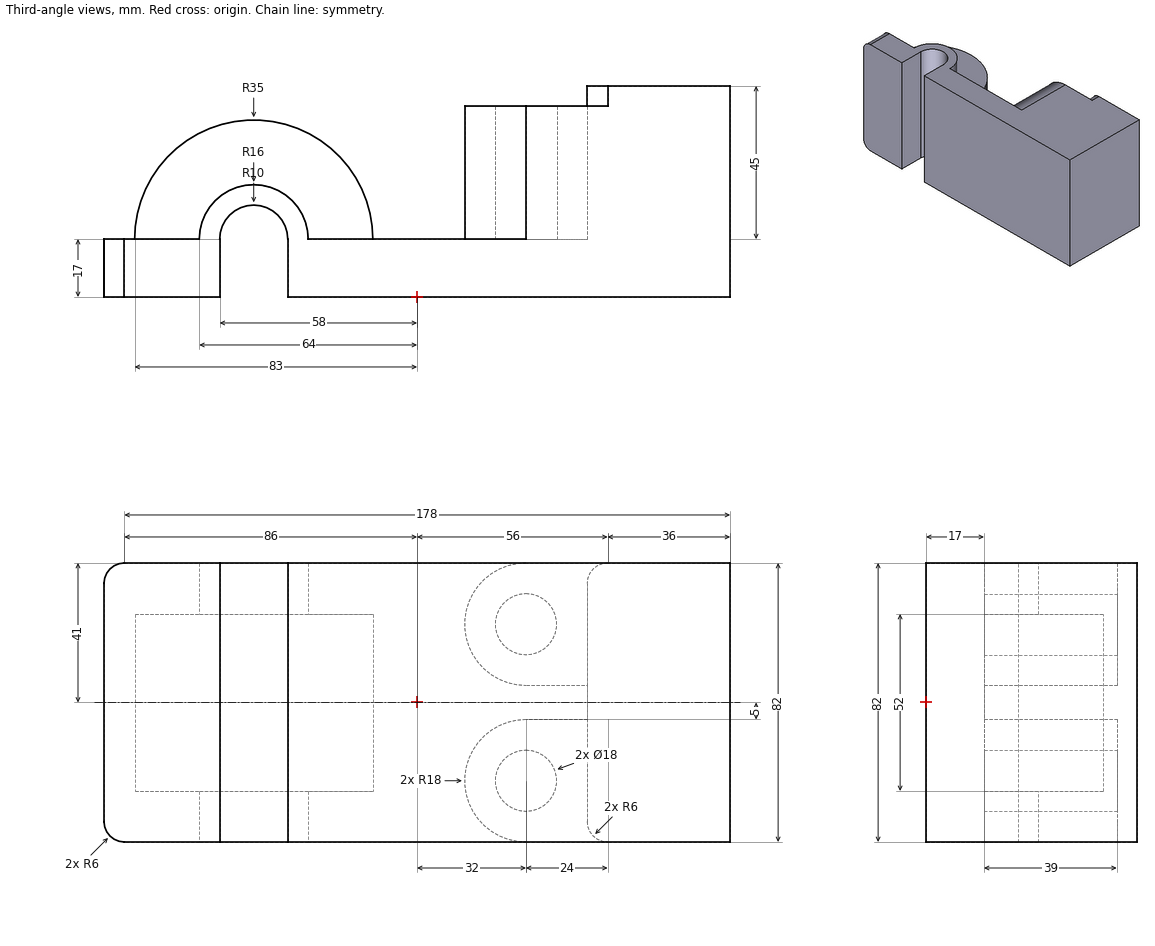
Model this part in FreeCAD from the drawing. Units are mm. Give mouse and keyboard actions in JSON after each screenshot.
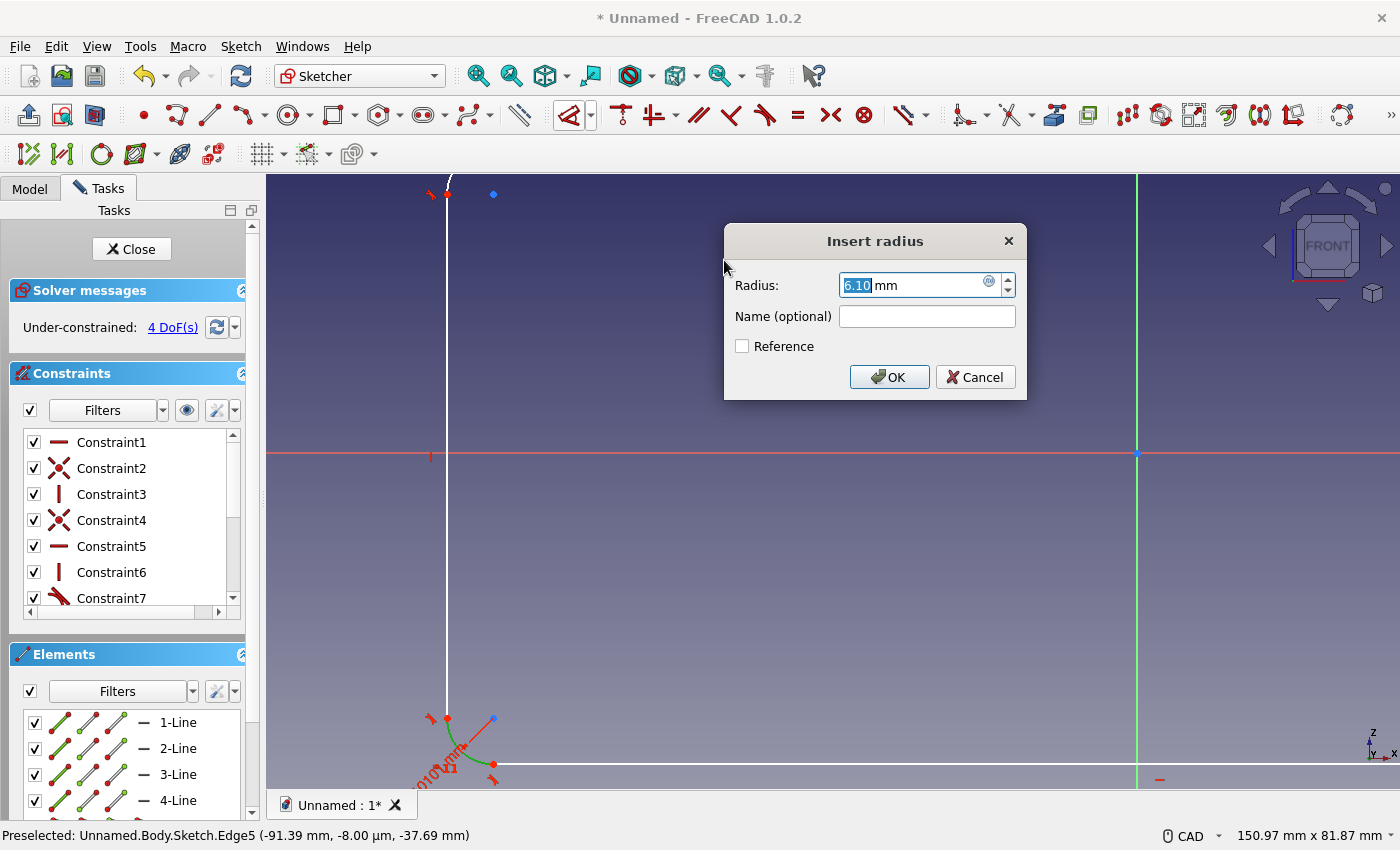
{"action": "type", "text": "6"}
{"action": "key", "text": "Return"}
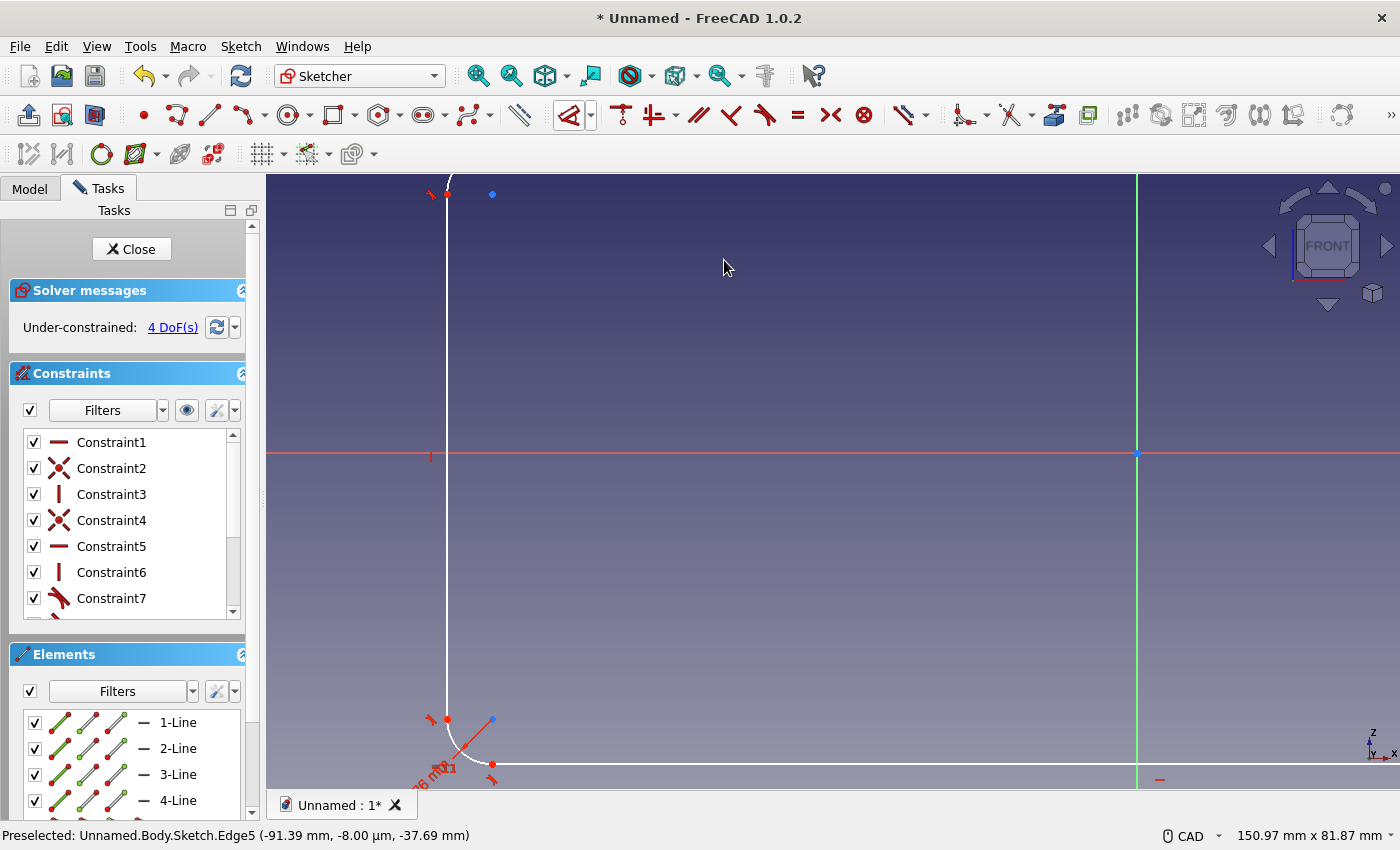
{"action": "scroll", "coordinate": [460, 504], "scroll_direction": "down", "scroll_amount": 4}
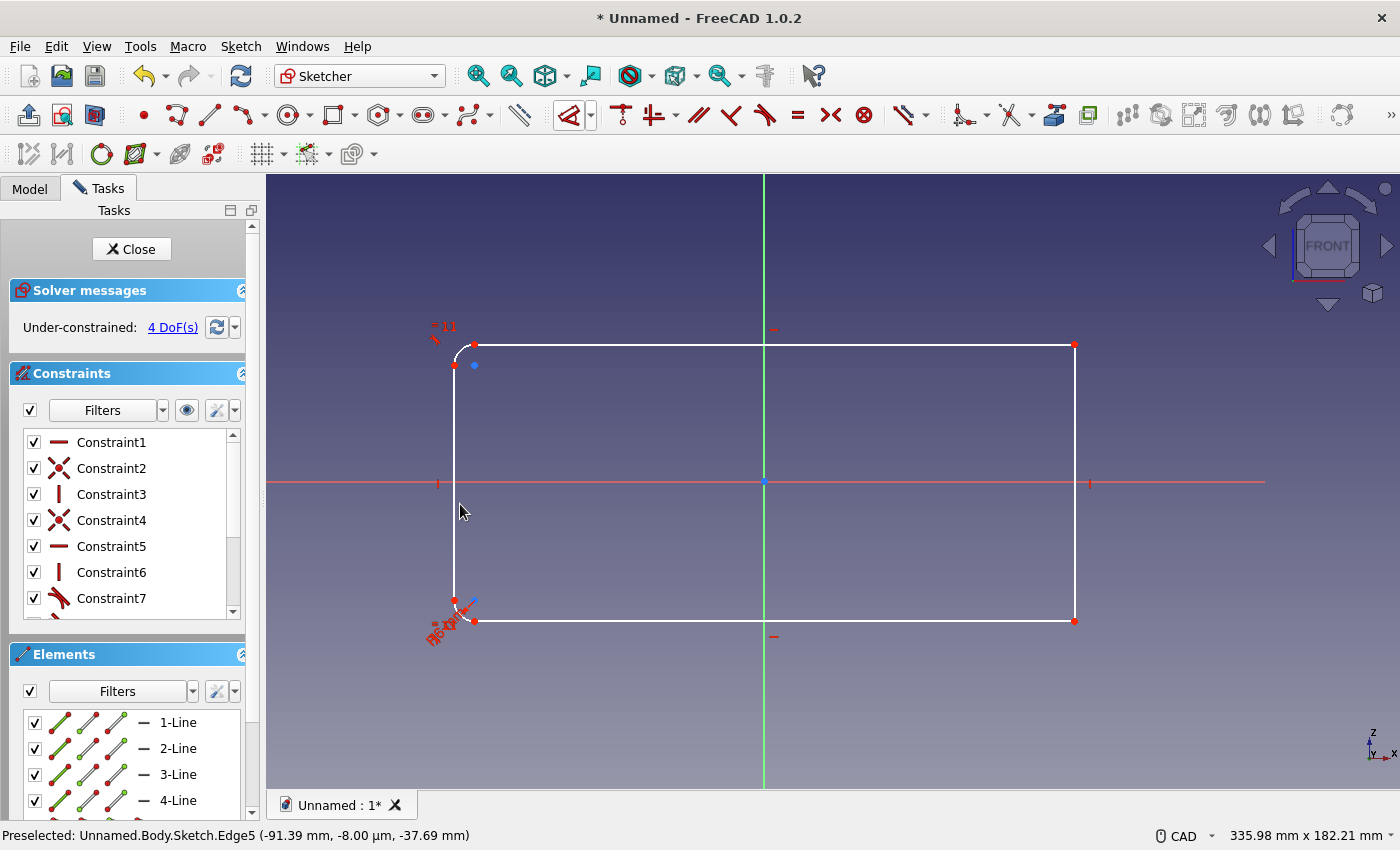
{"action": "left_click", "coordinate": [1075, 428]}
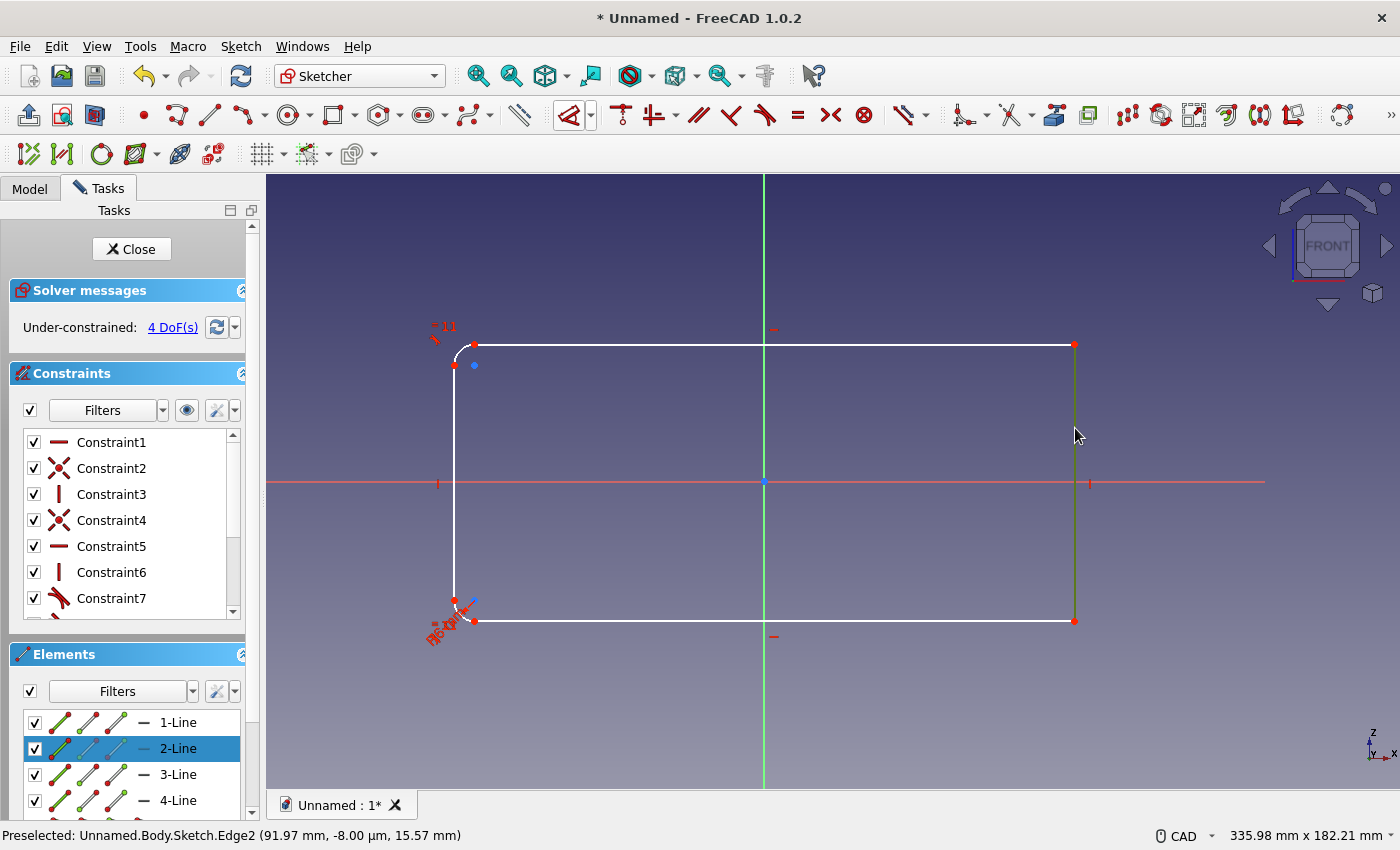
{"action": "left_click", "coordinate": [590, 116]}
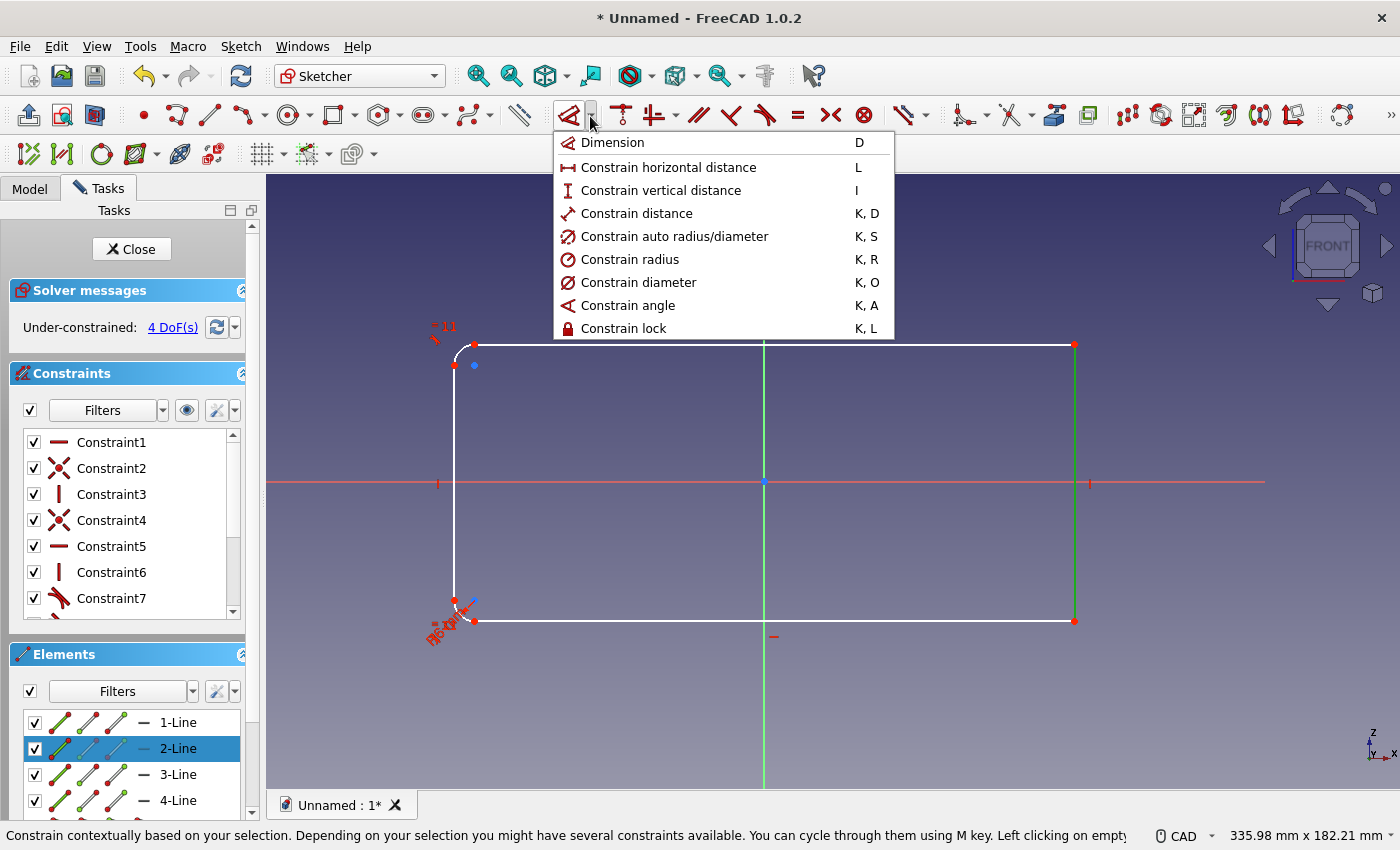
{"action": "left_click", "coordinate": [724, 190]}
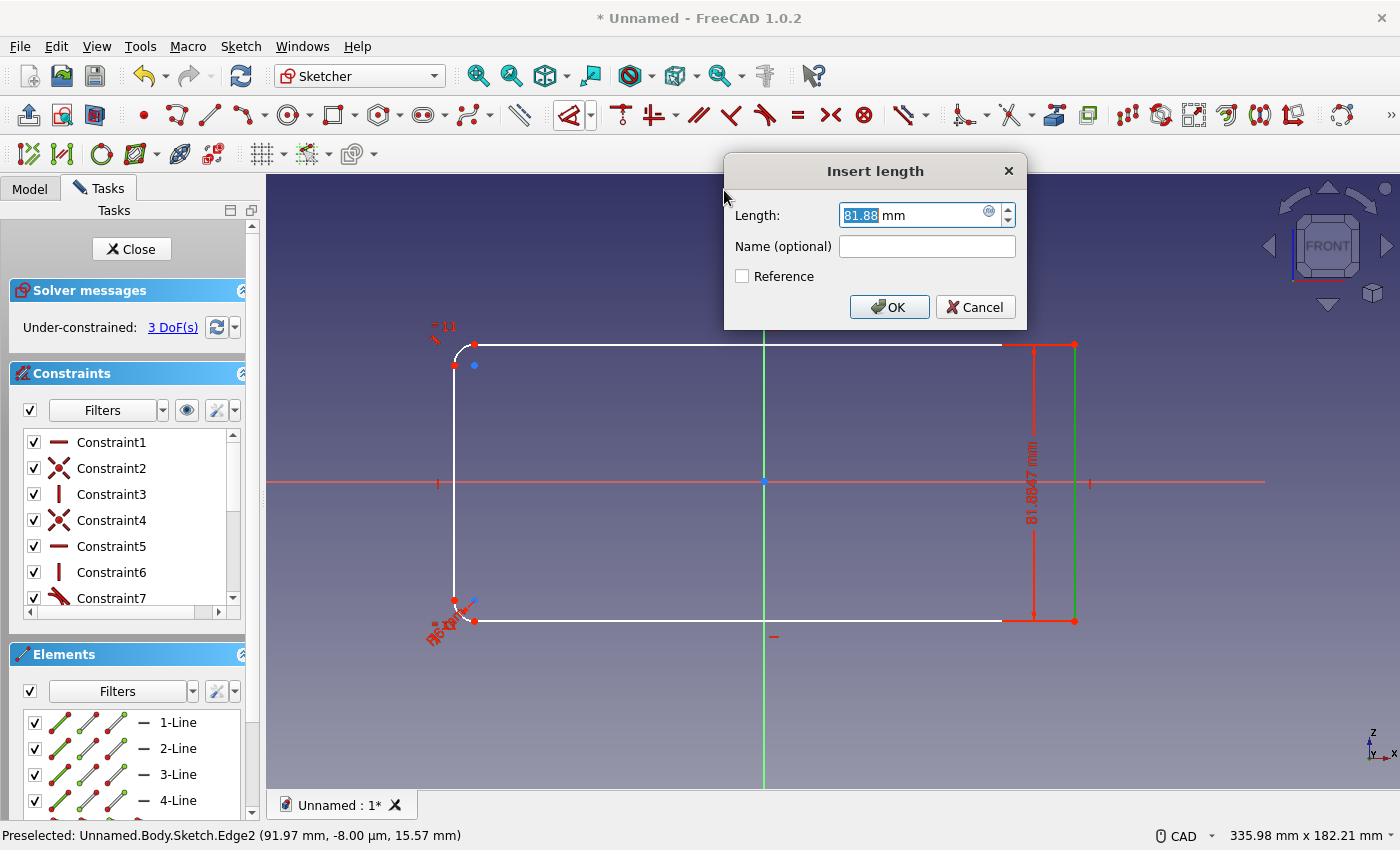
{"action": "type", "text": "82"}
{"action": "key", "text": "Return"}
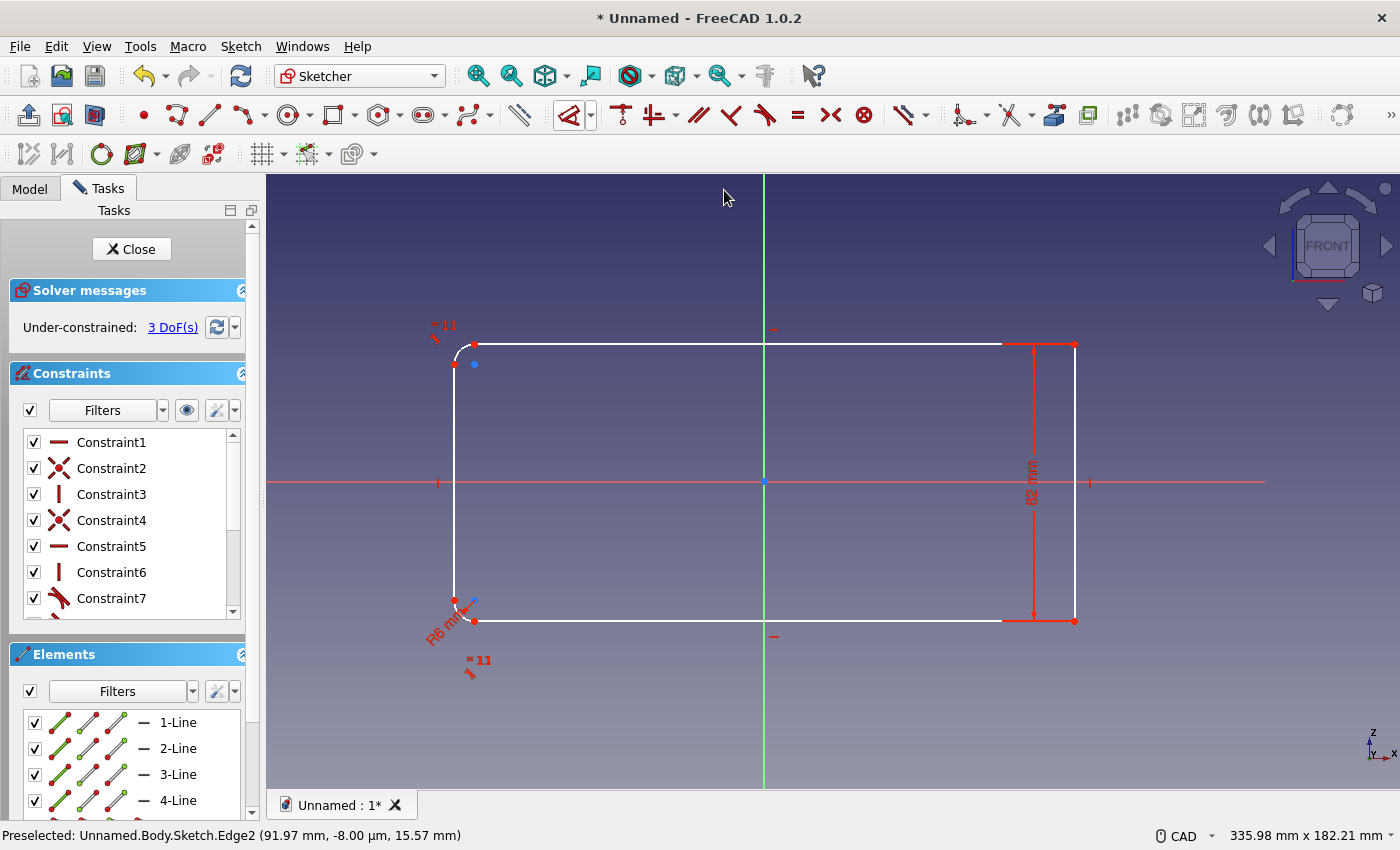
{"action": "left_click", "coordinate": [655, 344]}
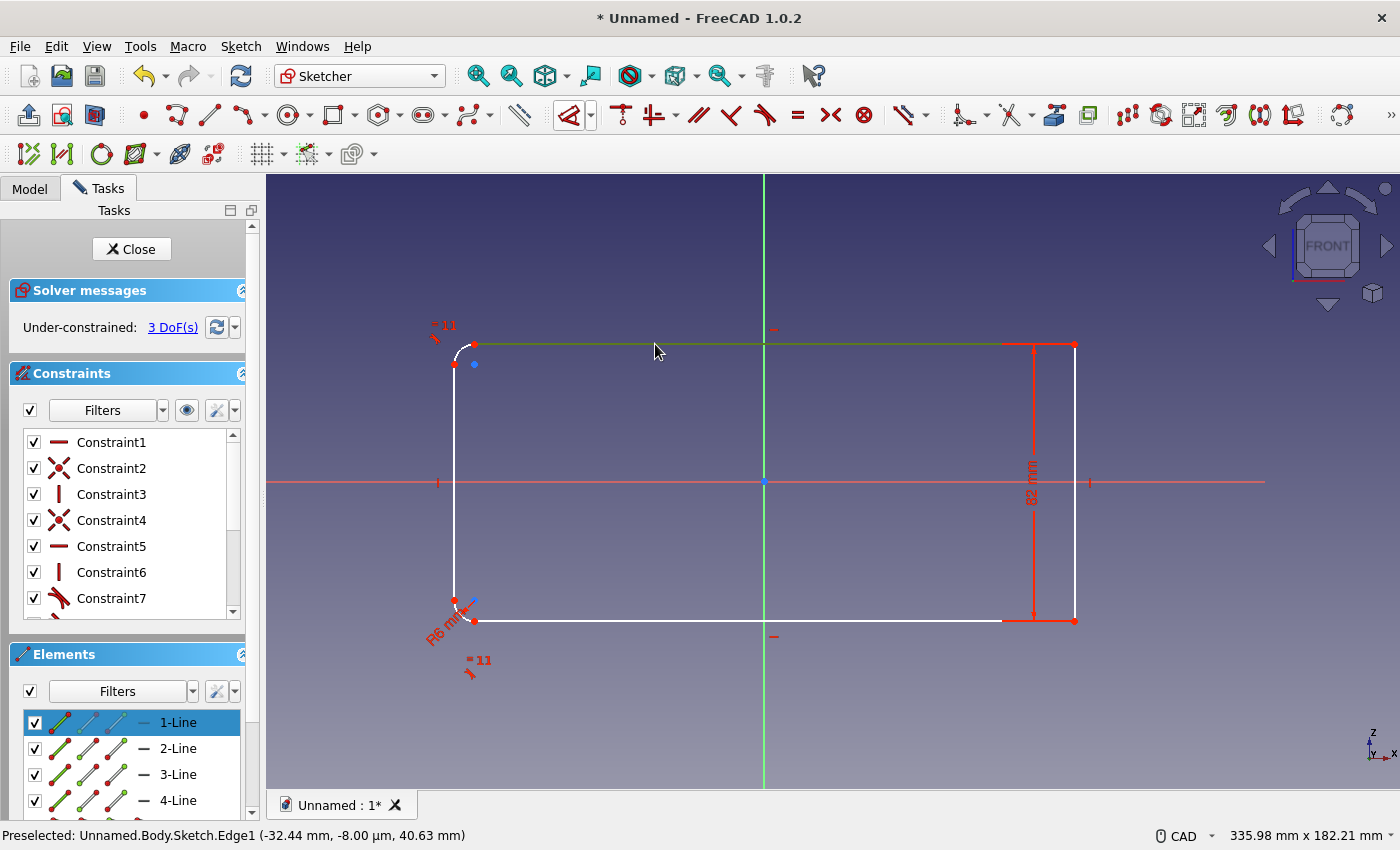
{"action": "left_click", "coordinate": [590, 116]}